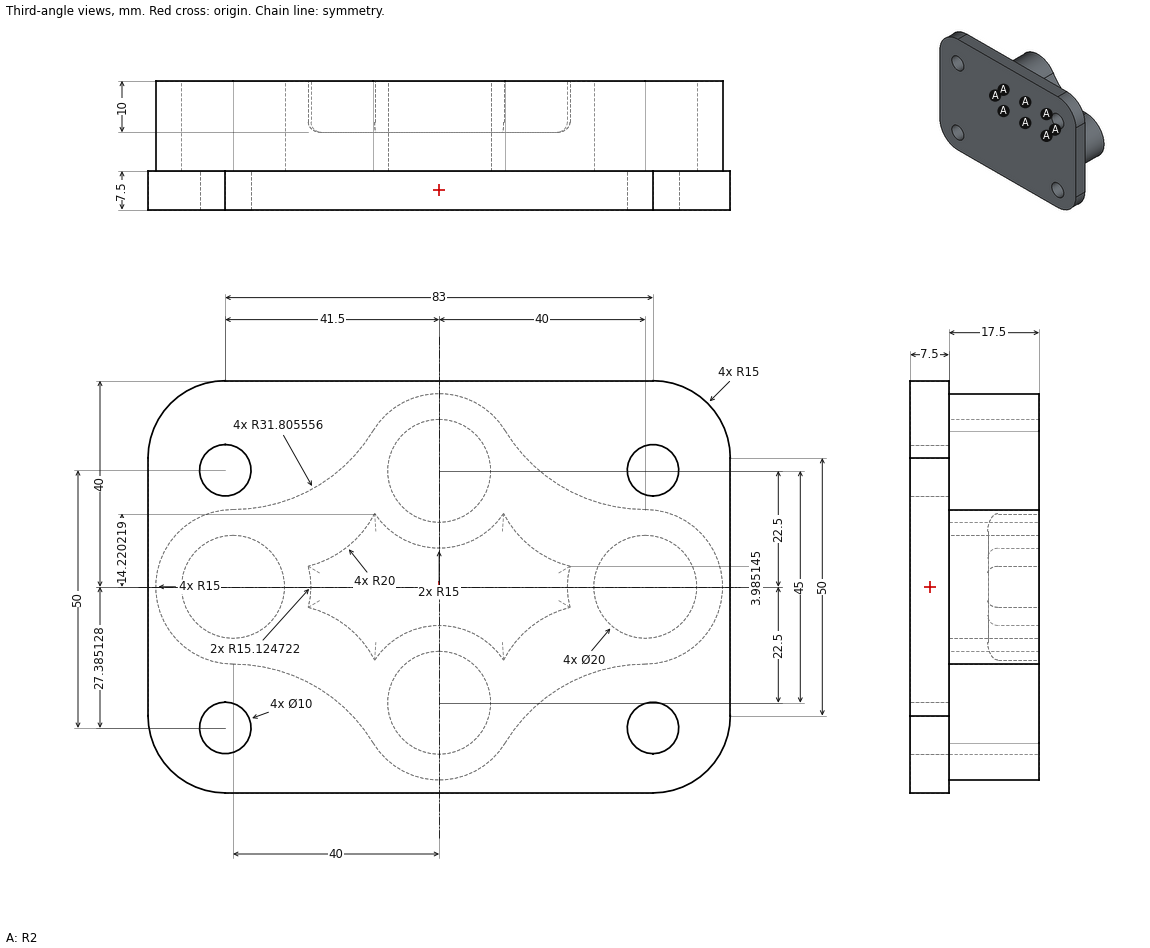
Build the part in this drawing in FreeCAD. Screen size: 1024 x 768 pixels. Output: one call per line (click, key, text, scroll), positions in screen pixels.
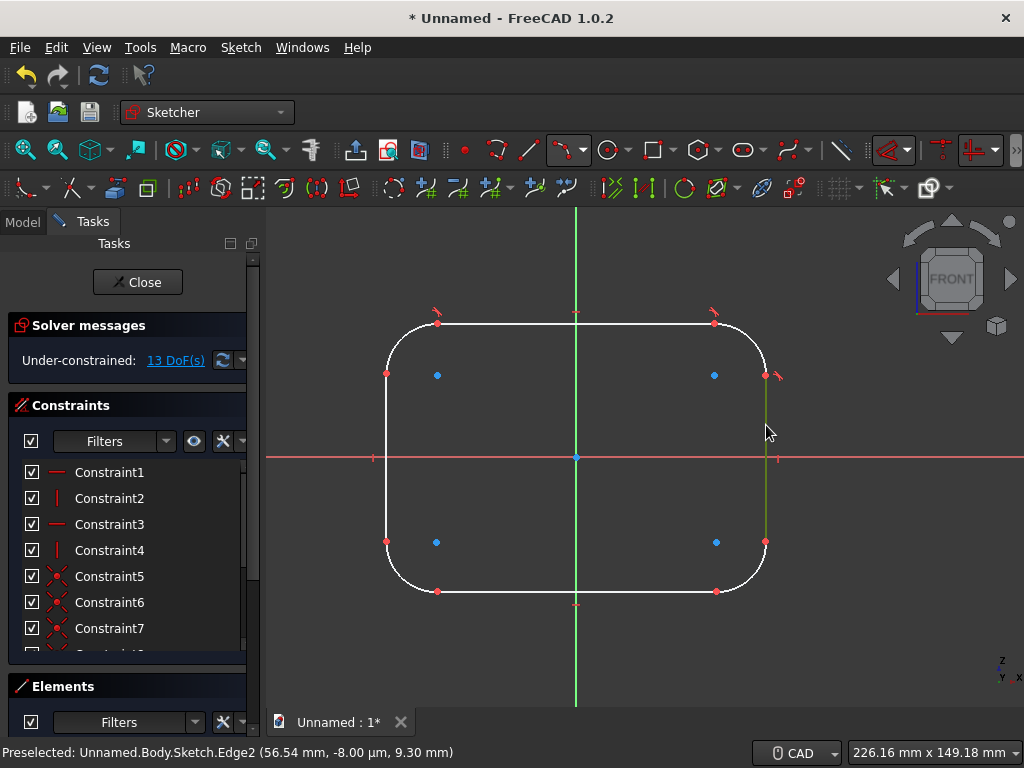
click(739, 587)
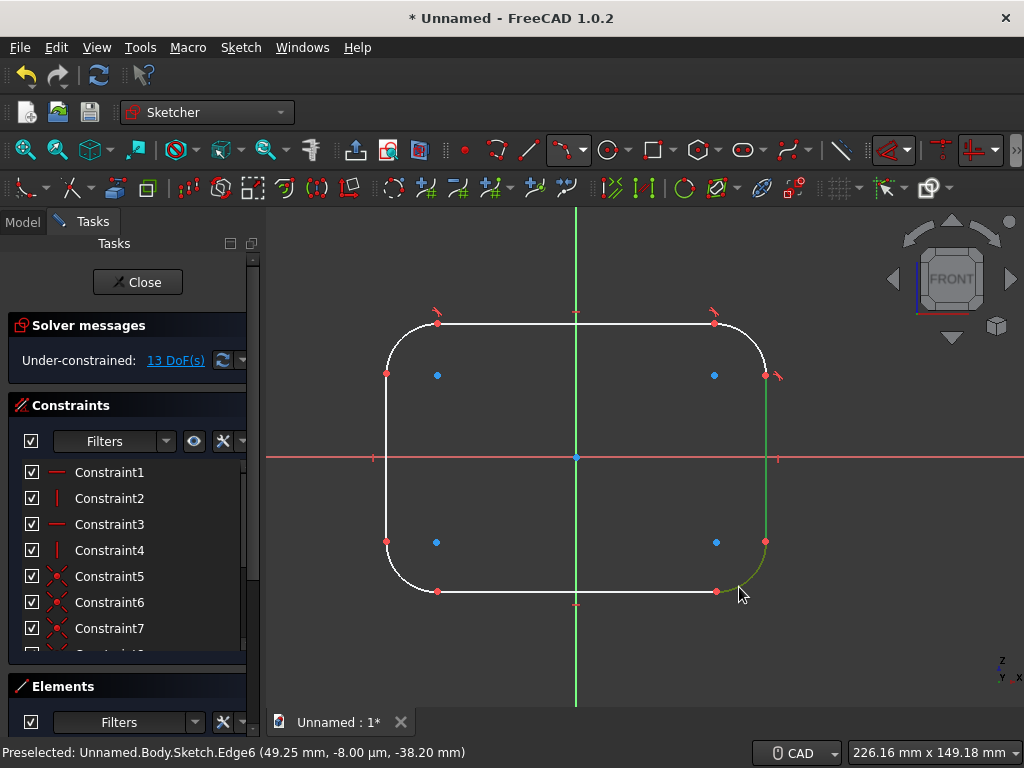
key(t)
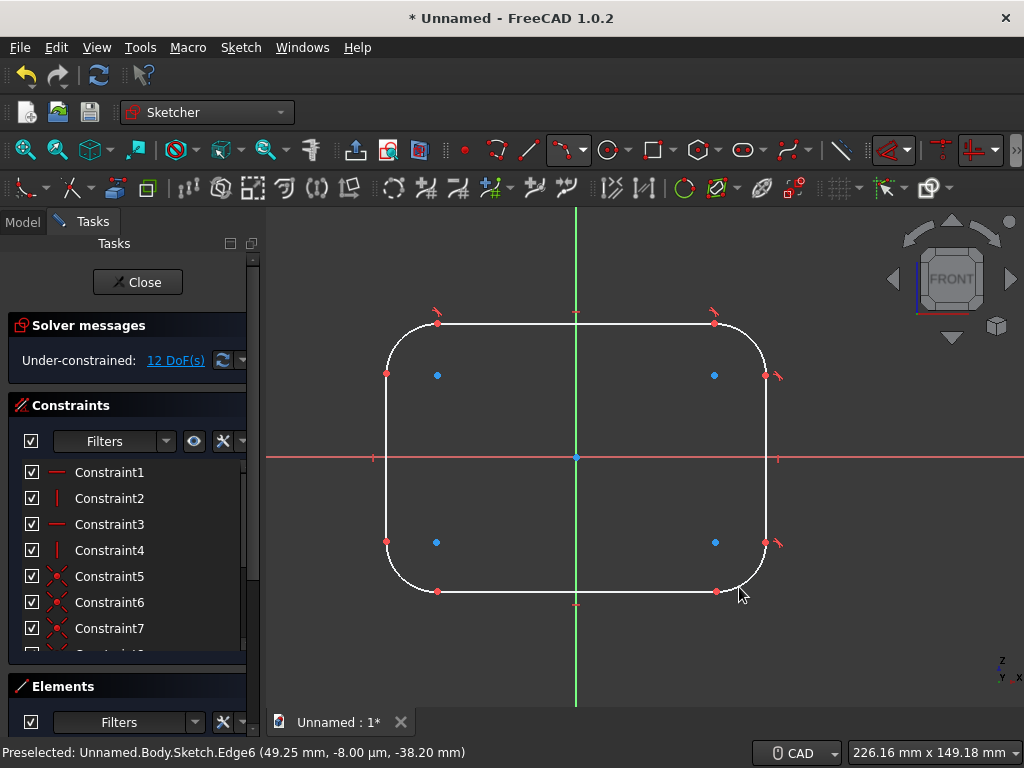
click(632, 592)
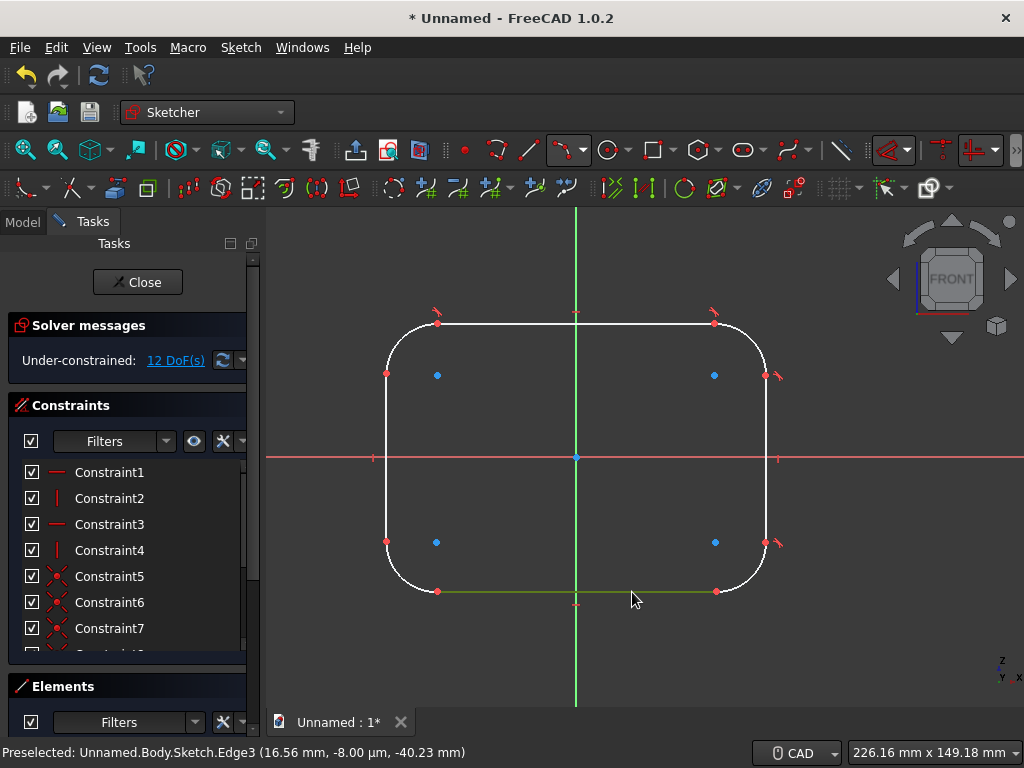
click(739, 587)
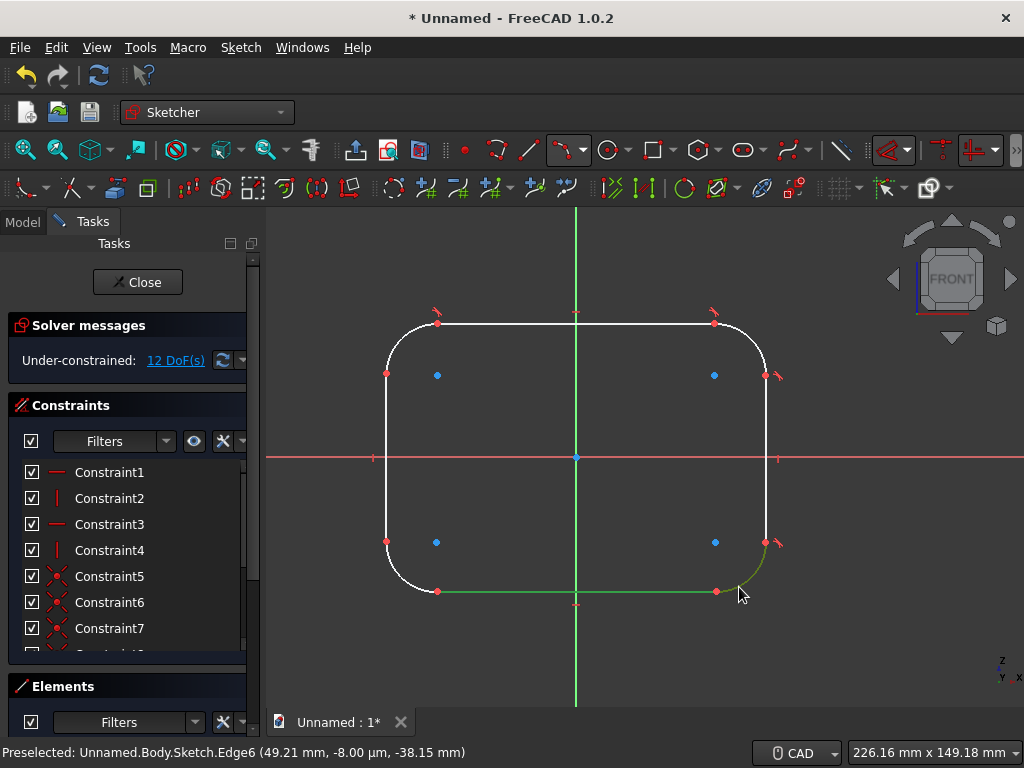
key(t)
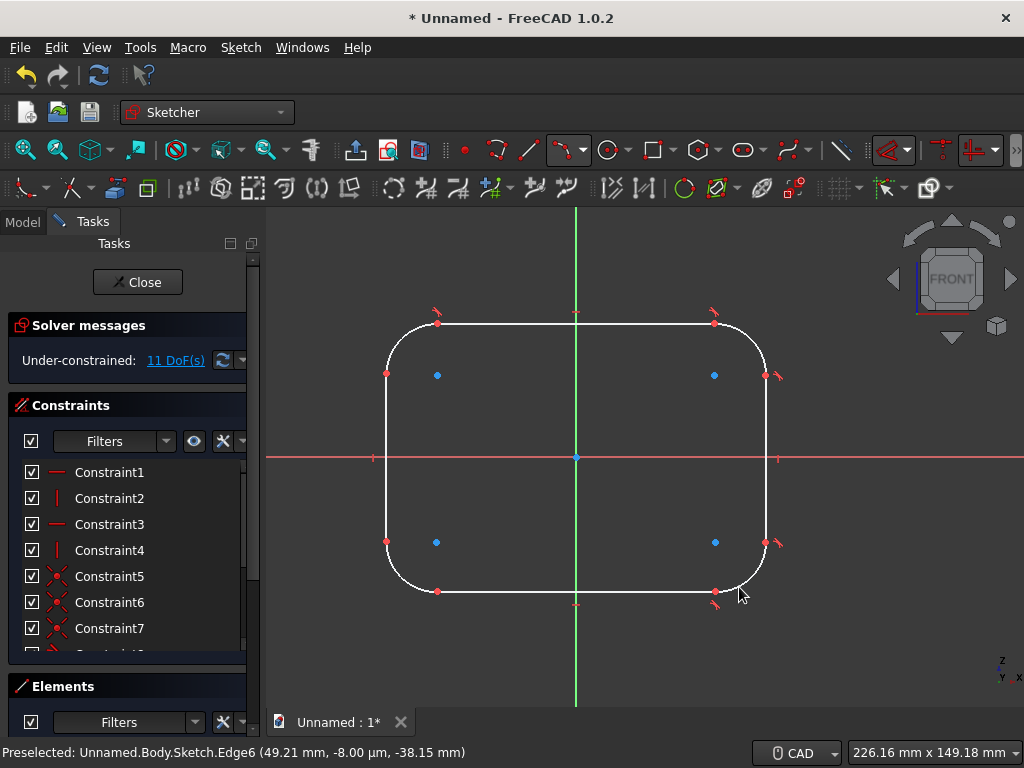
click(632, 592)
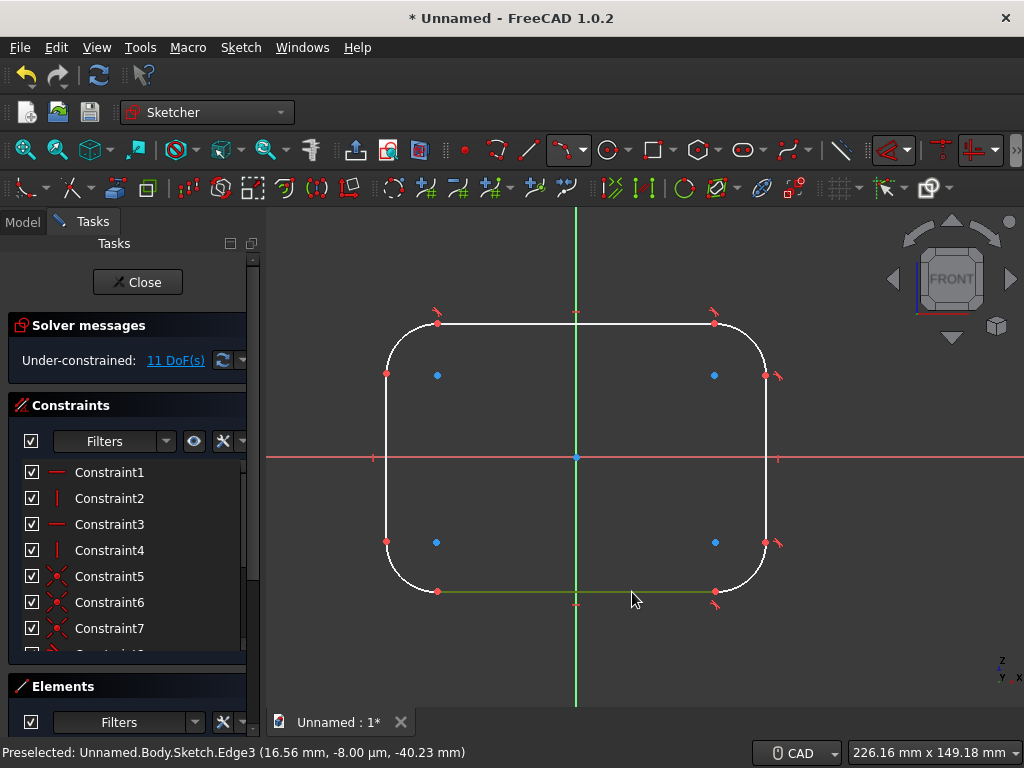
click(392, 565)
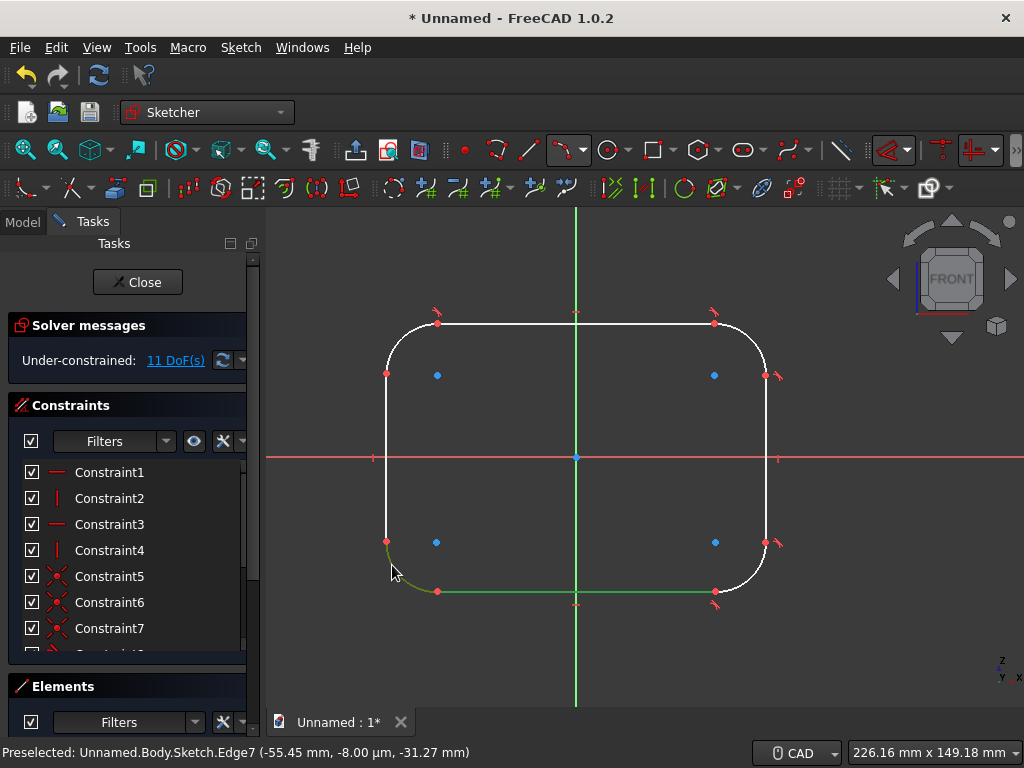
key(t)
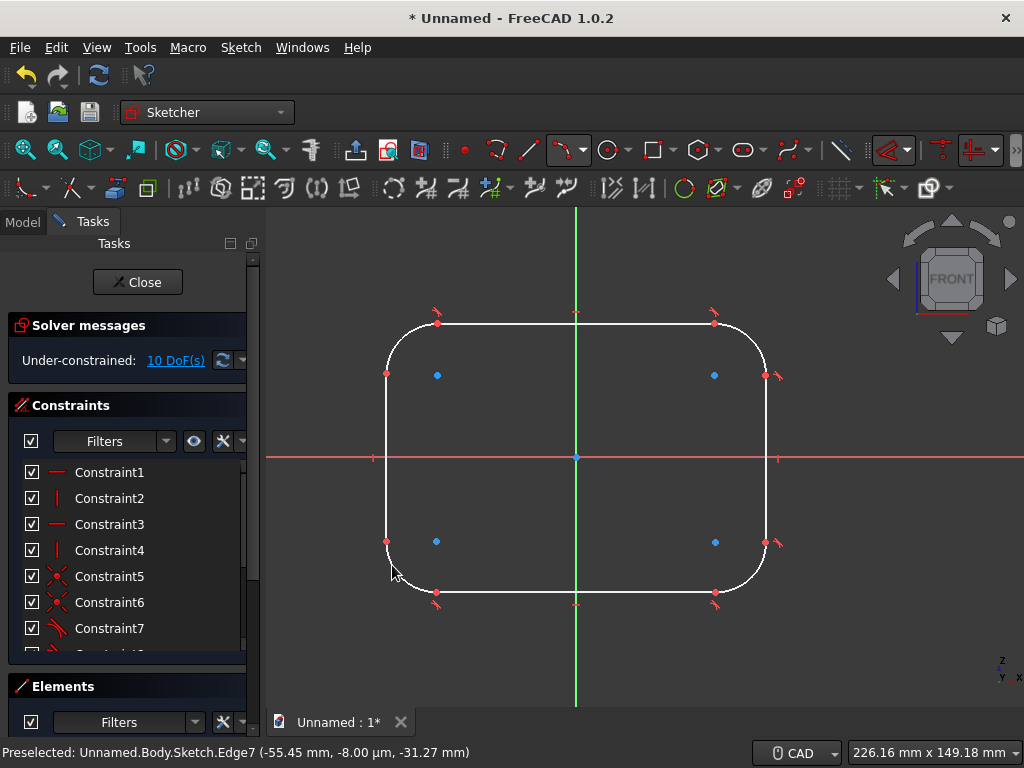
click(386, 492)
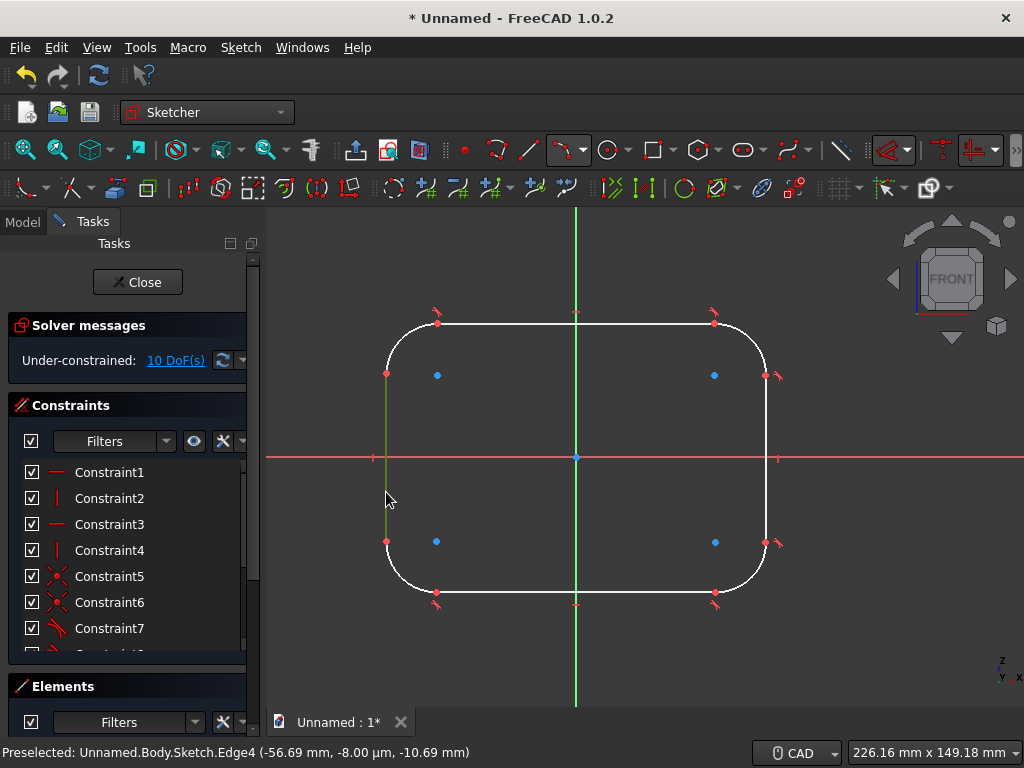
click(392, 565)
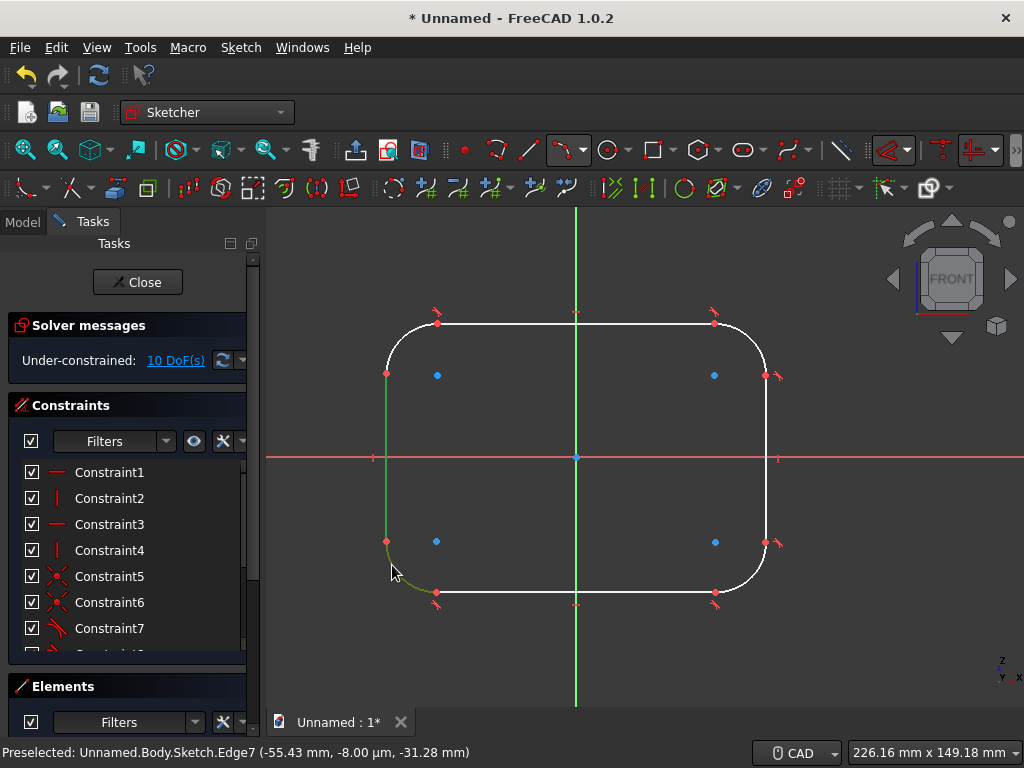
key(t)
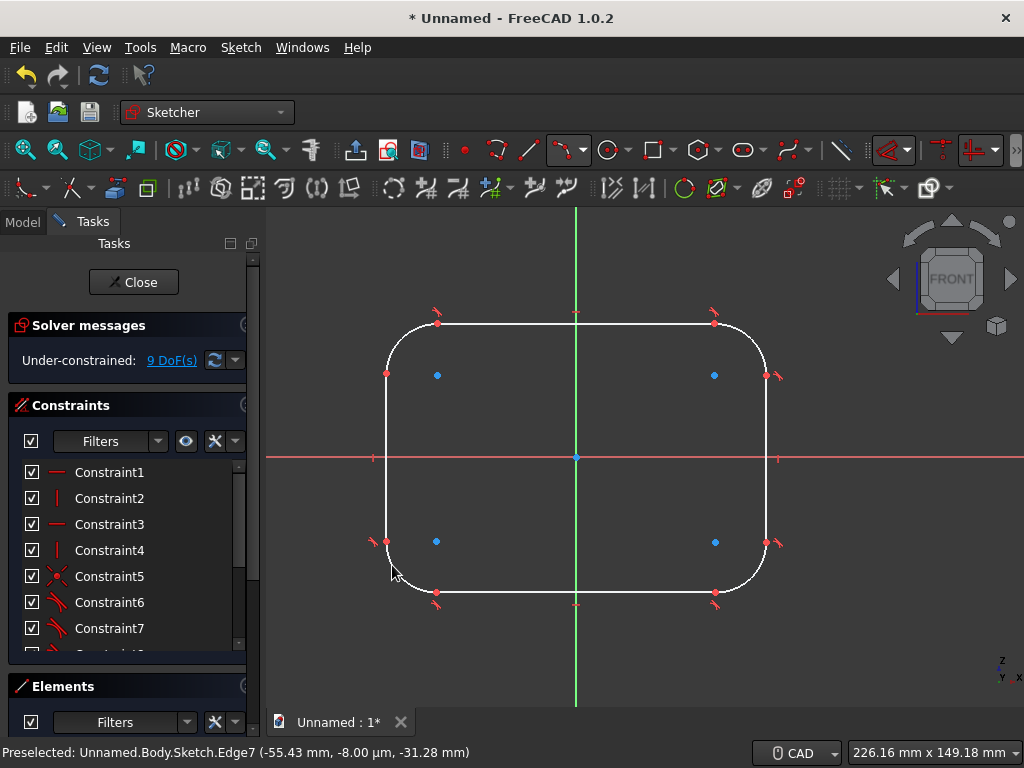
click(386, 492)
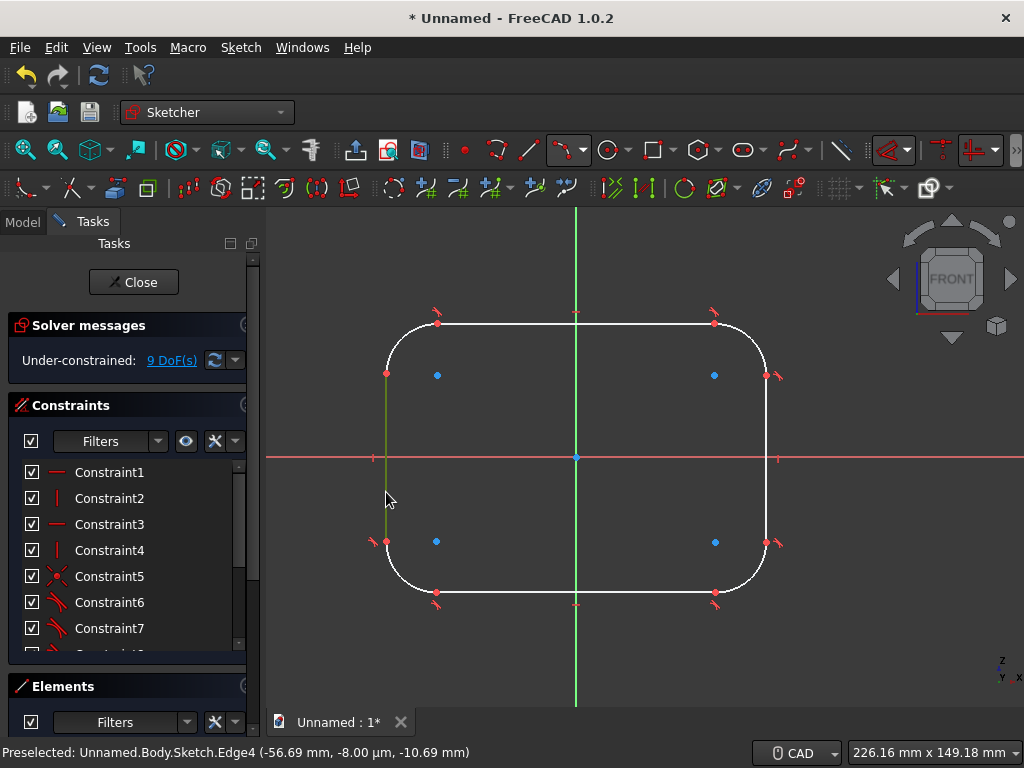
click(415, 329)